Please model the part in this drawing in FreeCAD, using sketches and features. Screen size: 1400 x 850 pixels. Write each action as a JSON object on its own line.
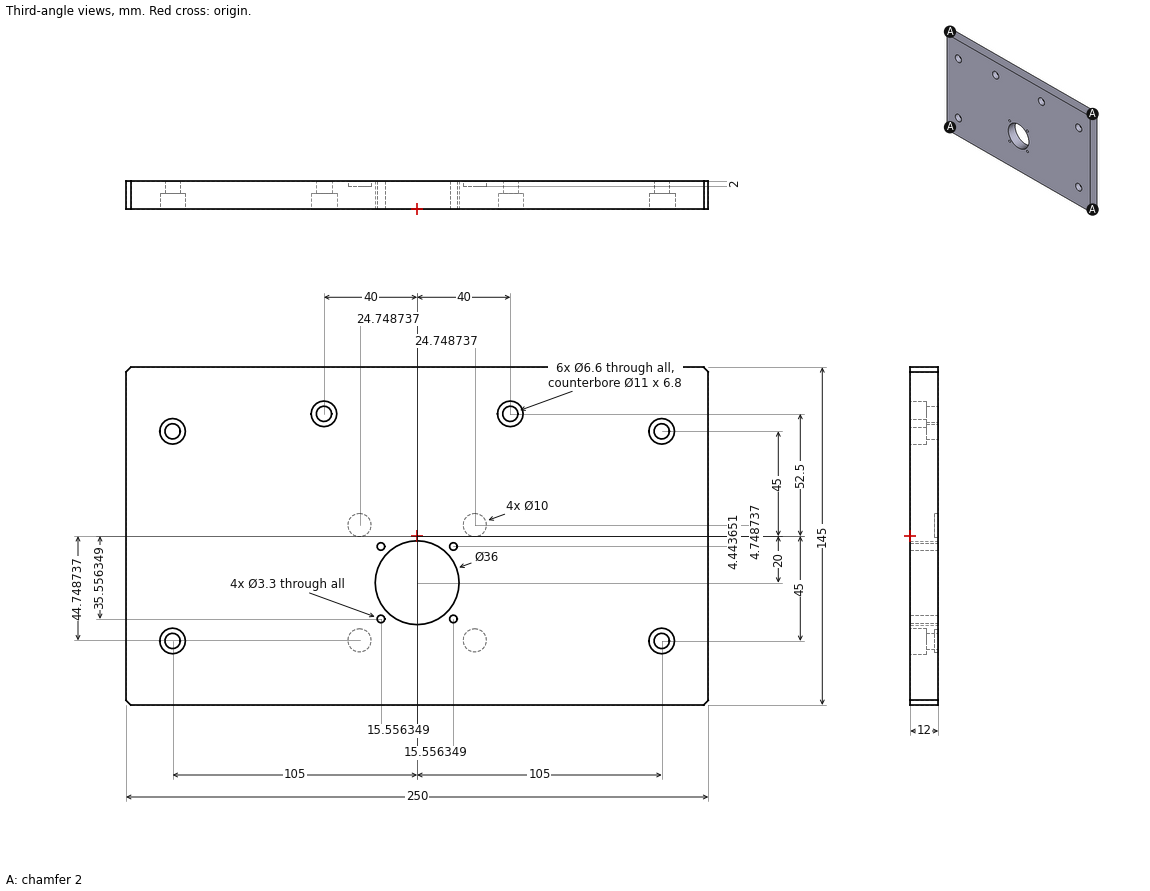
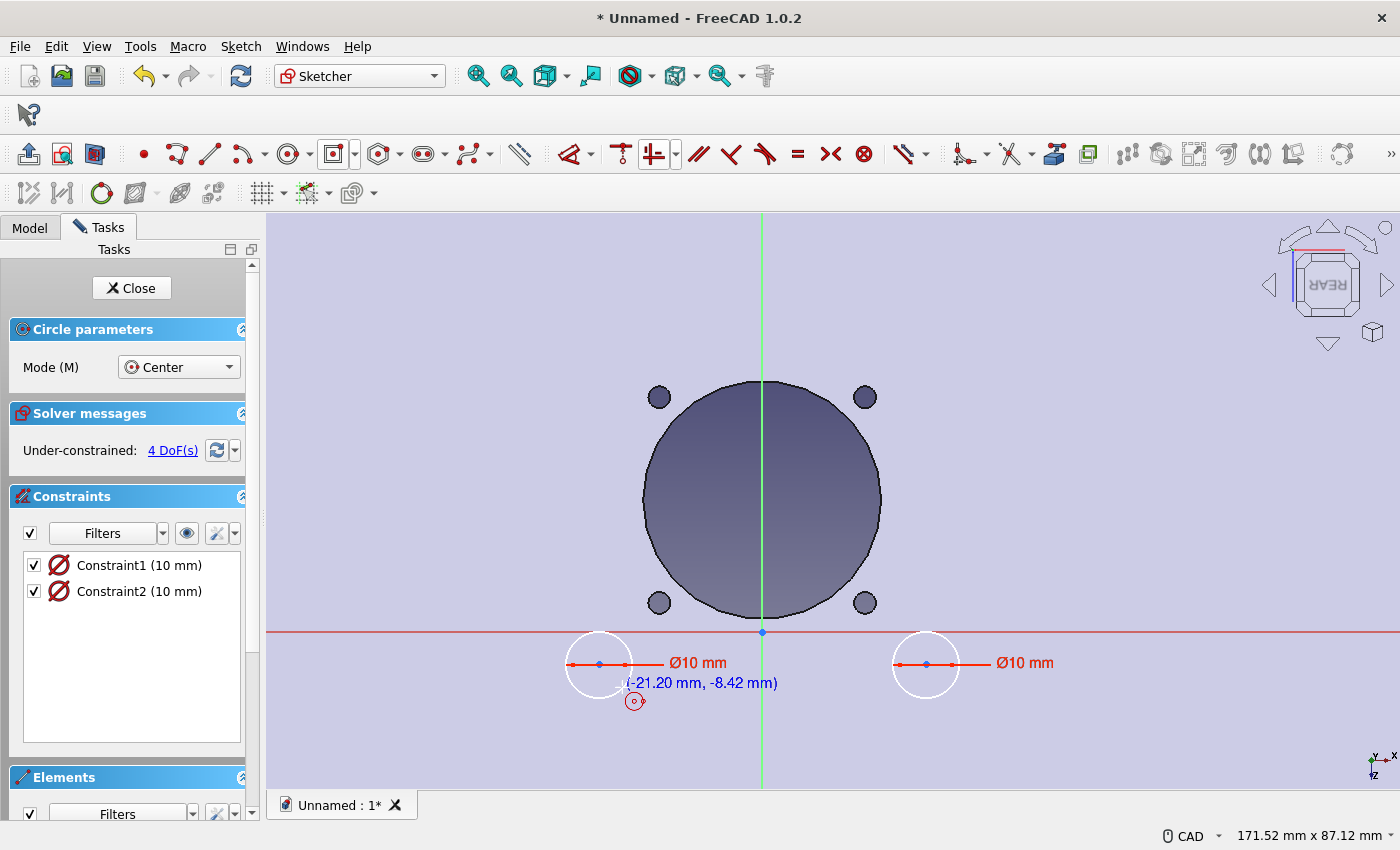
{"action": "left_click", "coordinate": [599, 336]}
{"action": "mouse_move", "coordinate": [622, 313]}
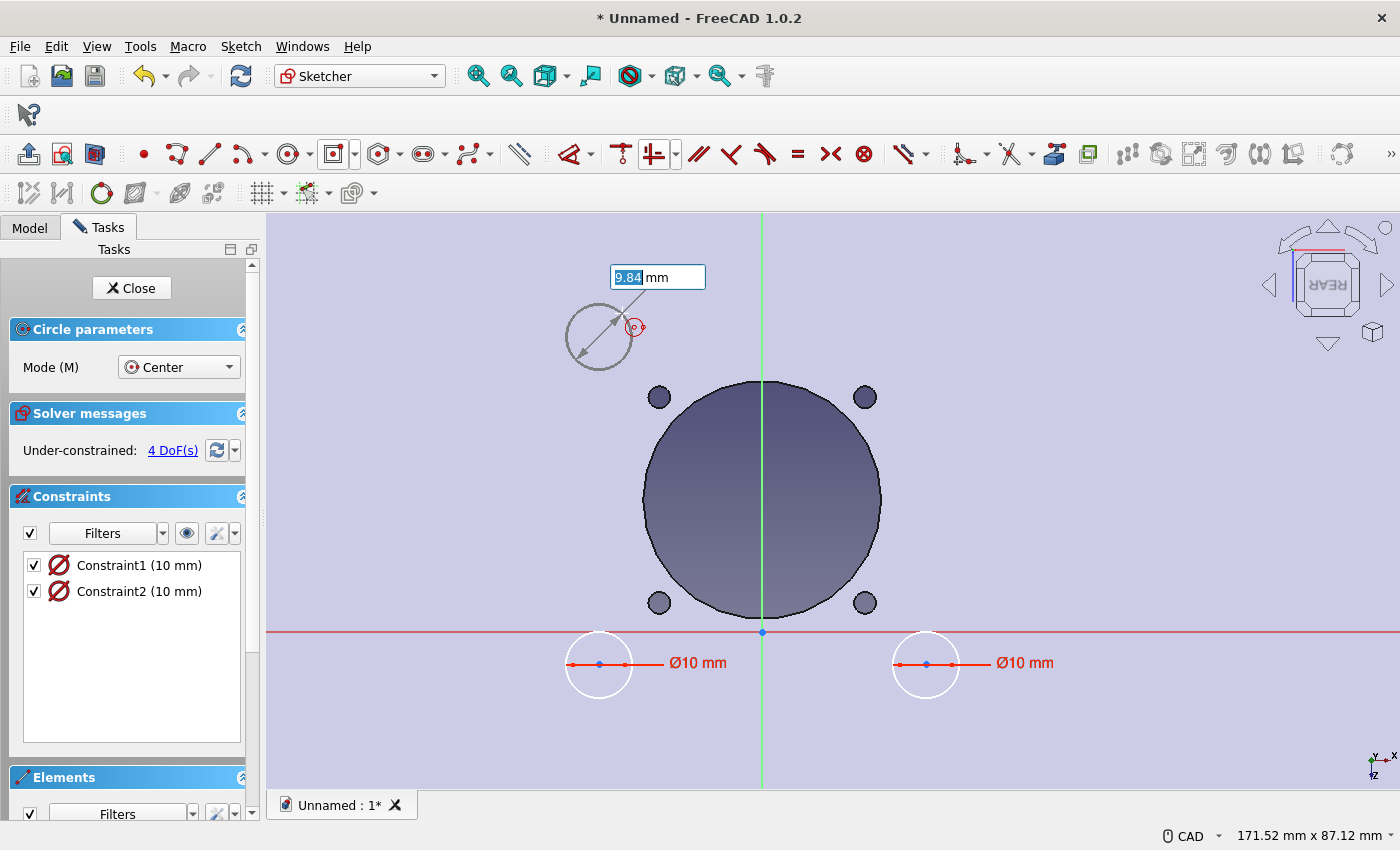
{"action": "type", "text": "10"}
{"action": "key", "text": "Return"}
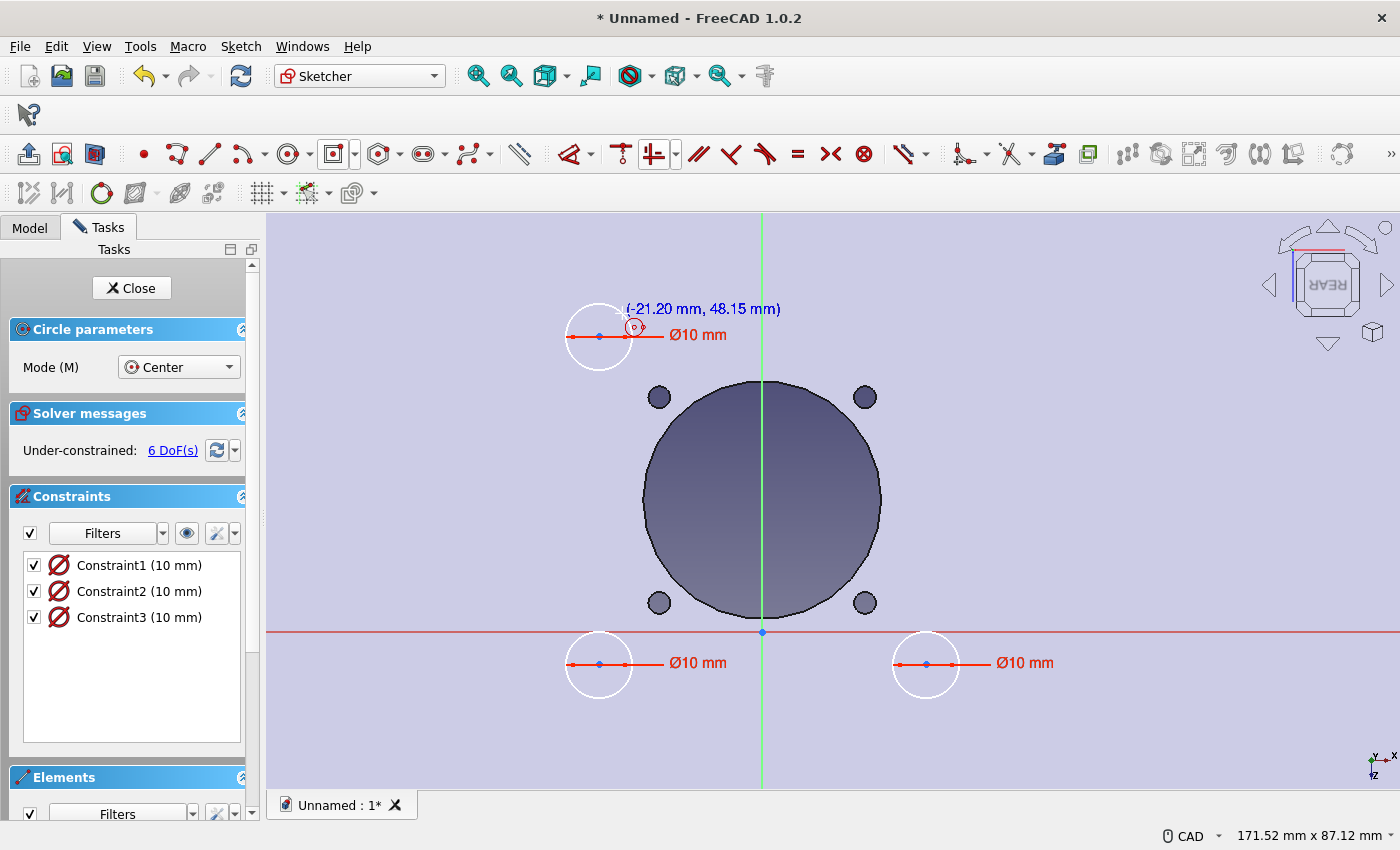
{"action": "left_click", "coordinate": [926, 336]}
{"action": "mouse_move", "coordinate": [949, 313]}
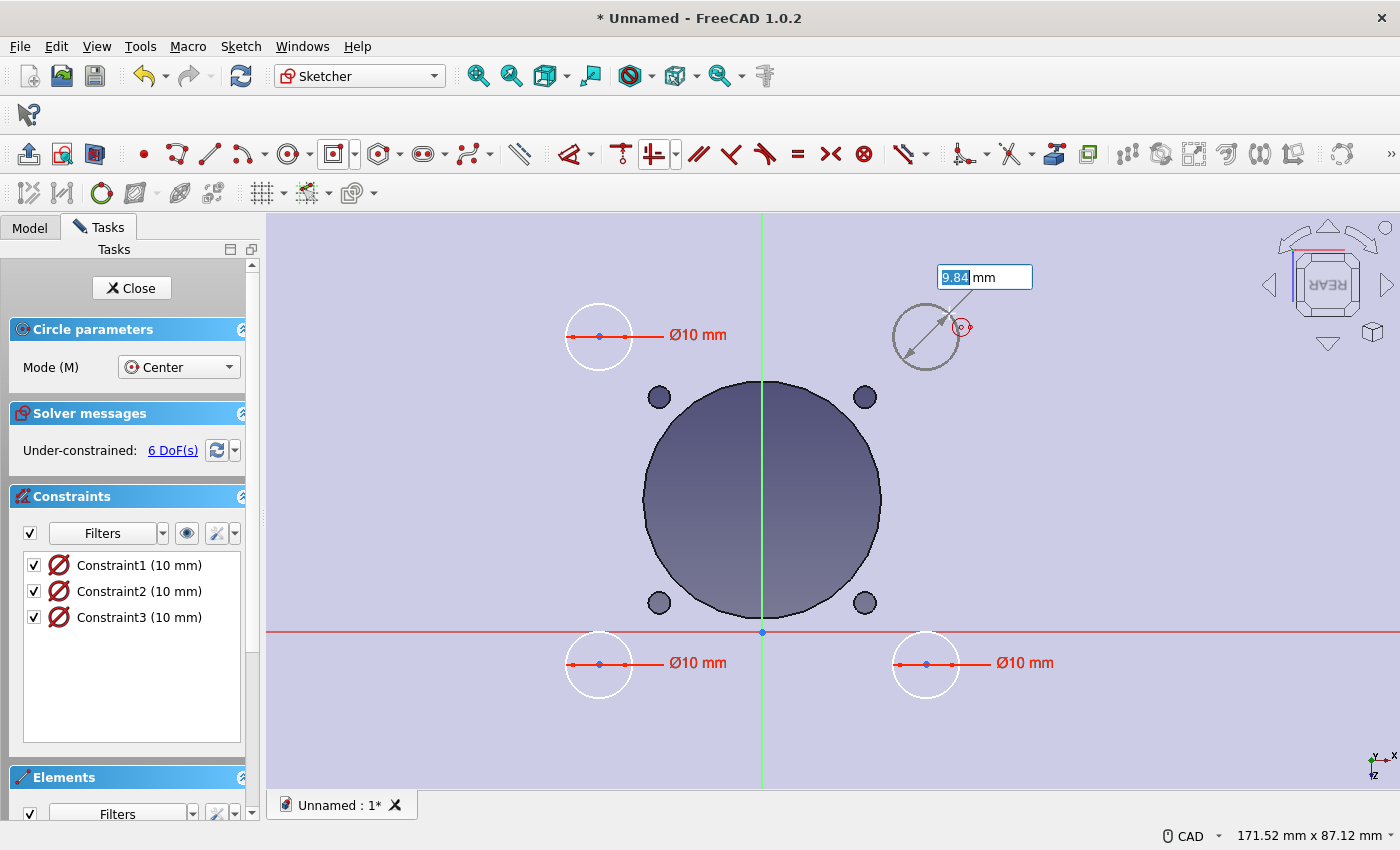
{"action": "type", "text": "10"}
{"action": "key", "text": "Return"}
{"action": "key", "text": "Escape"}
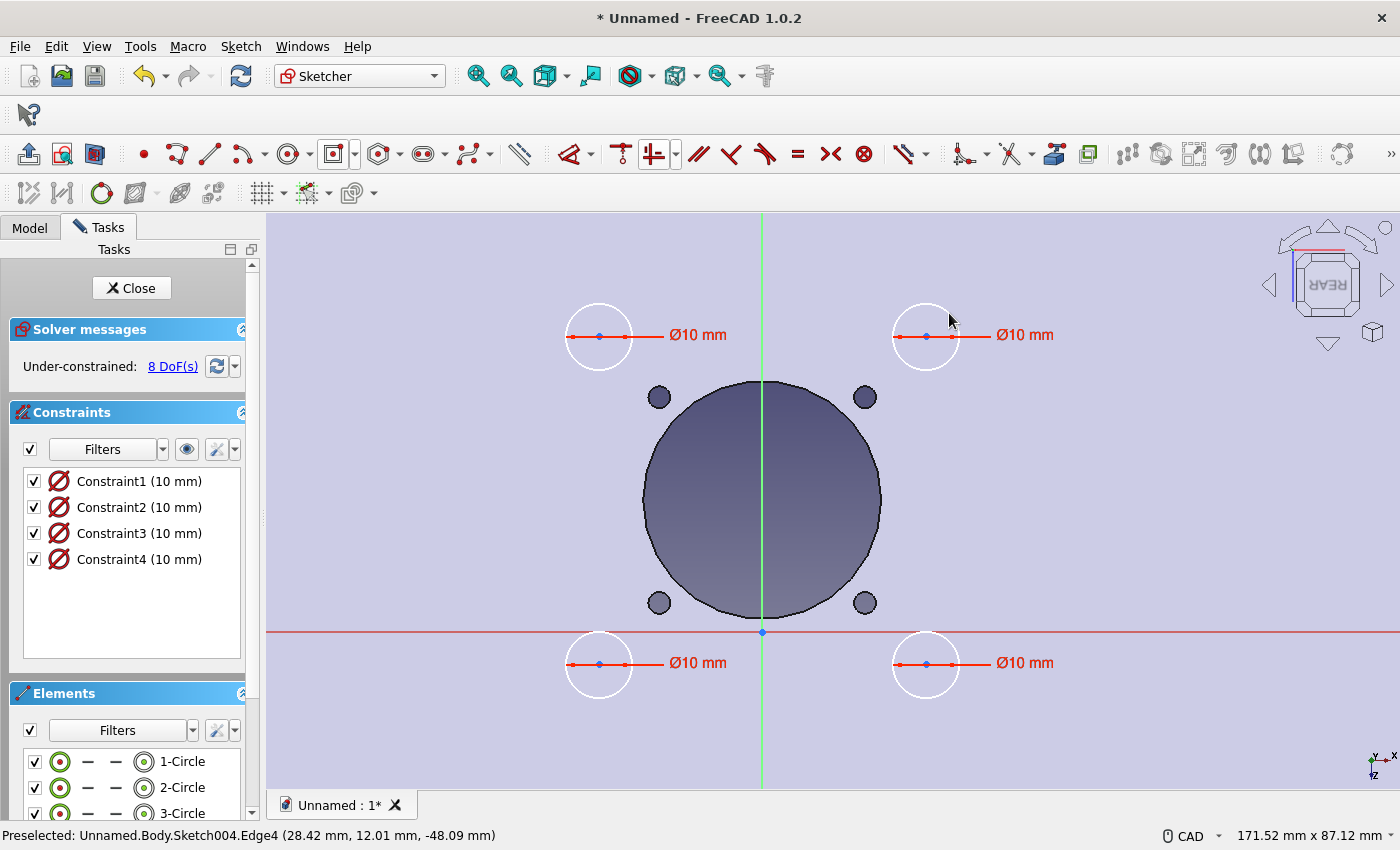
{"action": "left_click", "coordinate": [926, 665]}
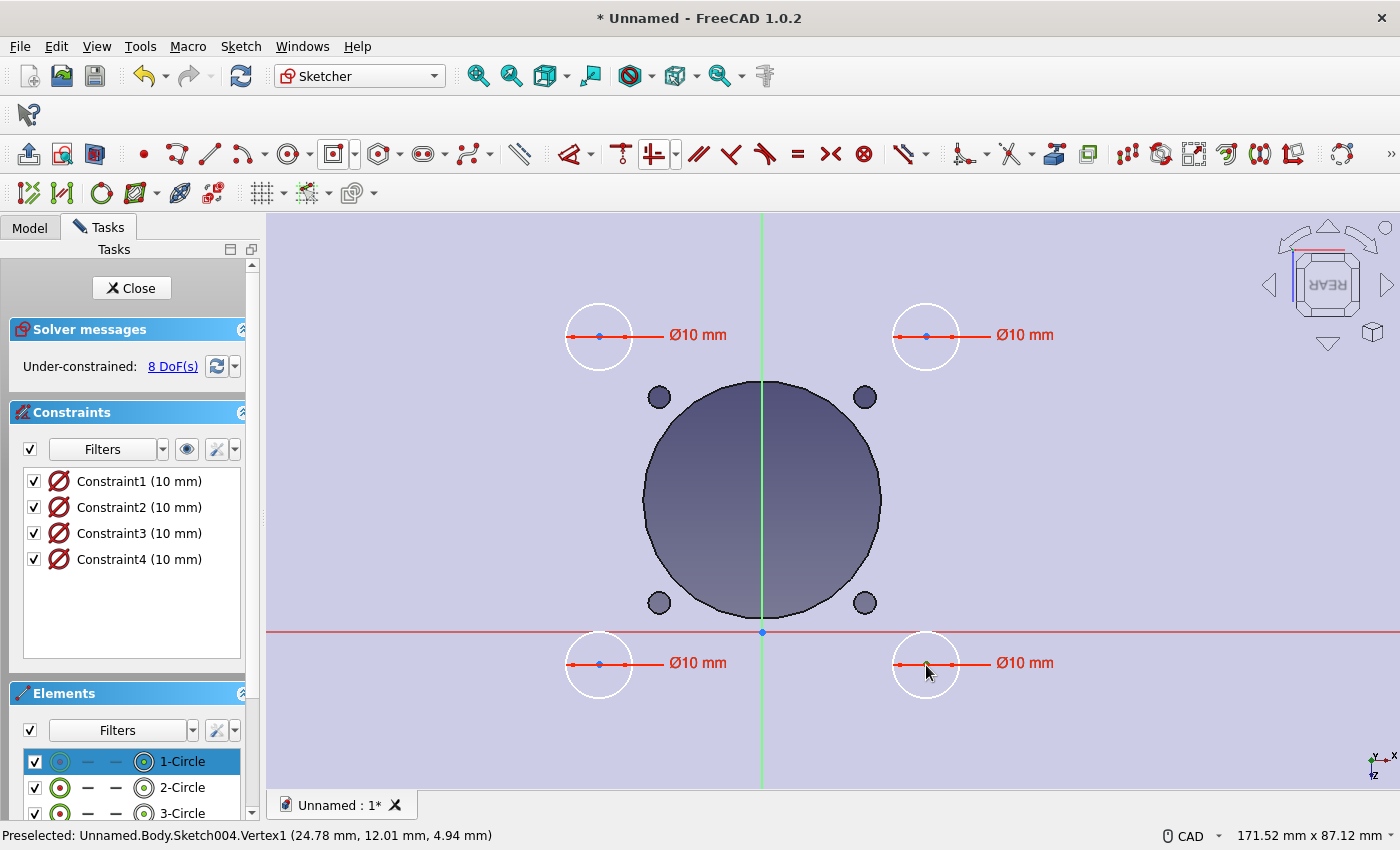
{"action": "left_click", "coordinate": [599, 665]}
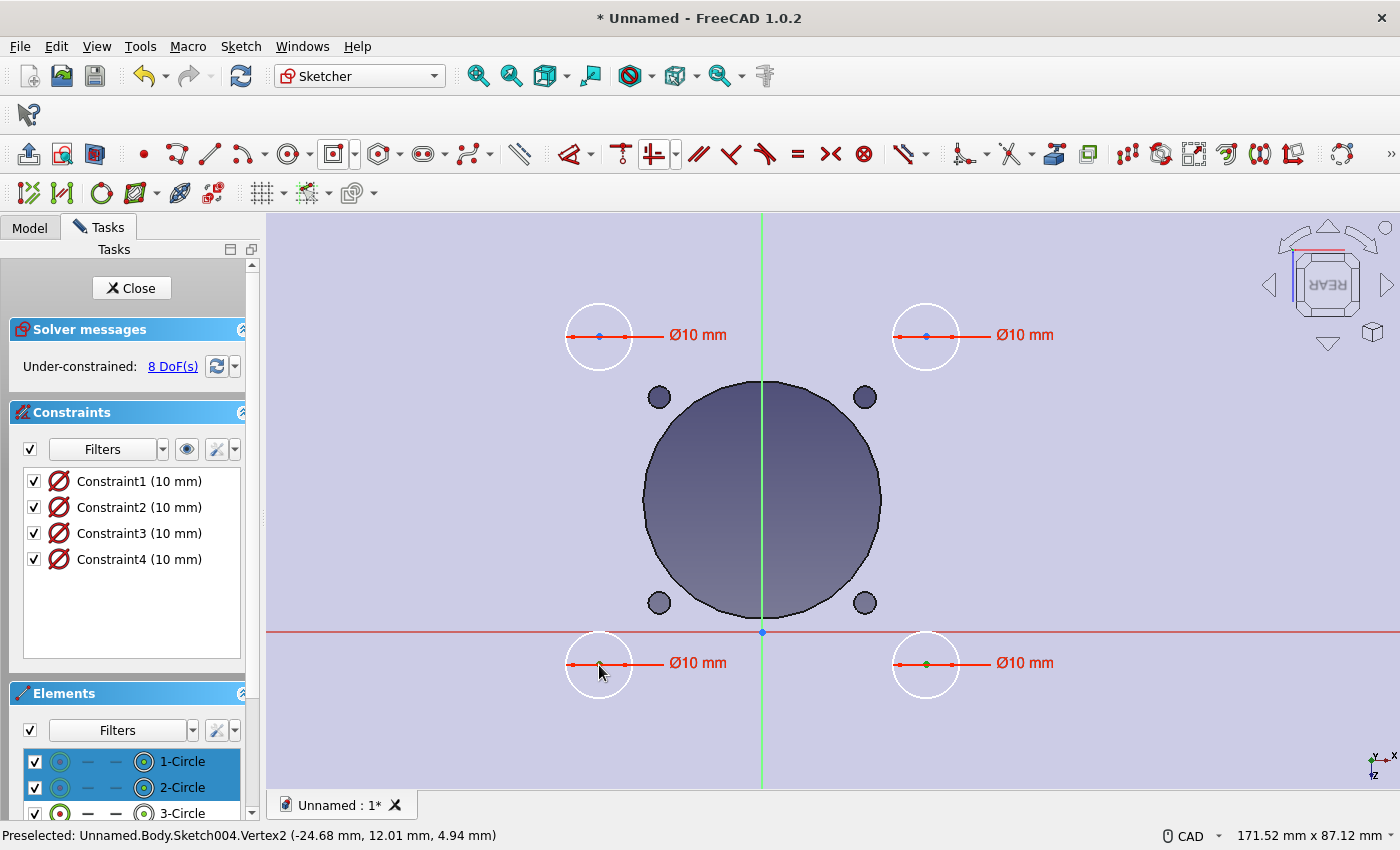
{"action": "left_click", "coordinate": [676, 154]}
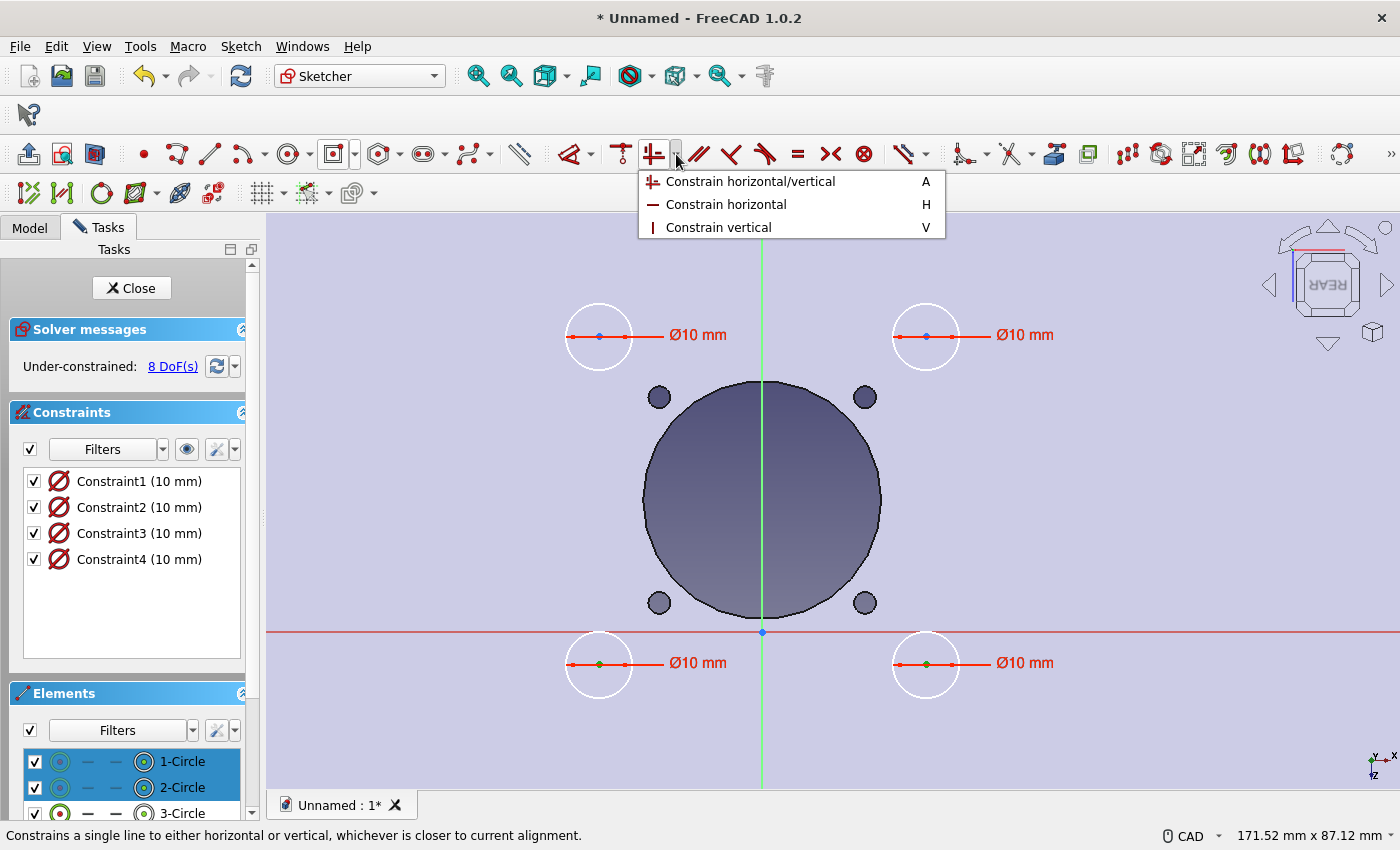
{"action": "left_click", "coordinate": [792, 204]}